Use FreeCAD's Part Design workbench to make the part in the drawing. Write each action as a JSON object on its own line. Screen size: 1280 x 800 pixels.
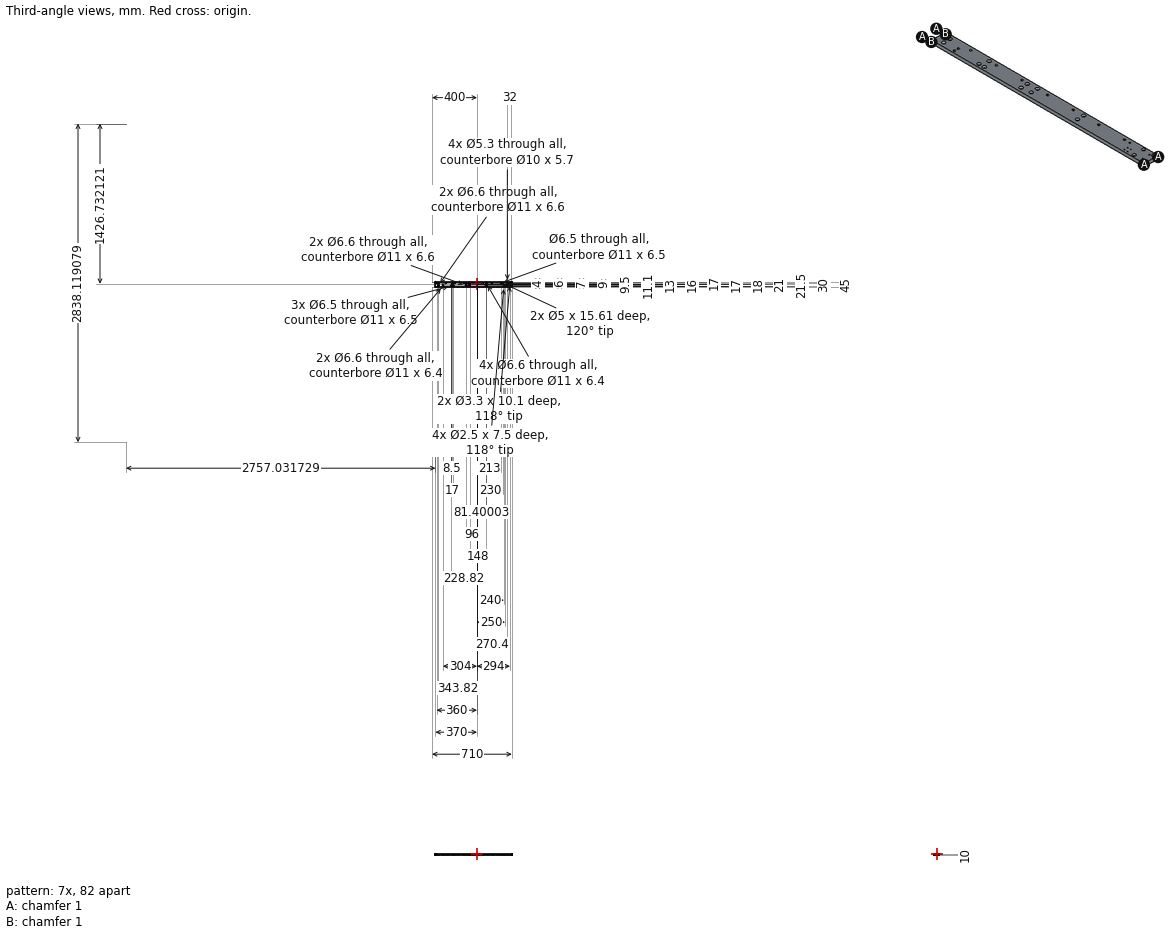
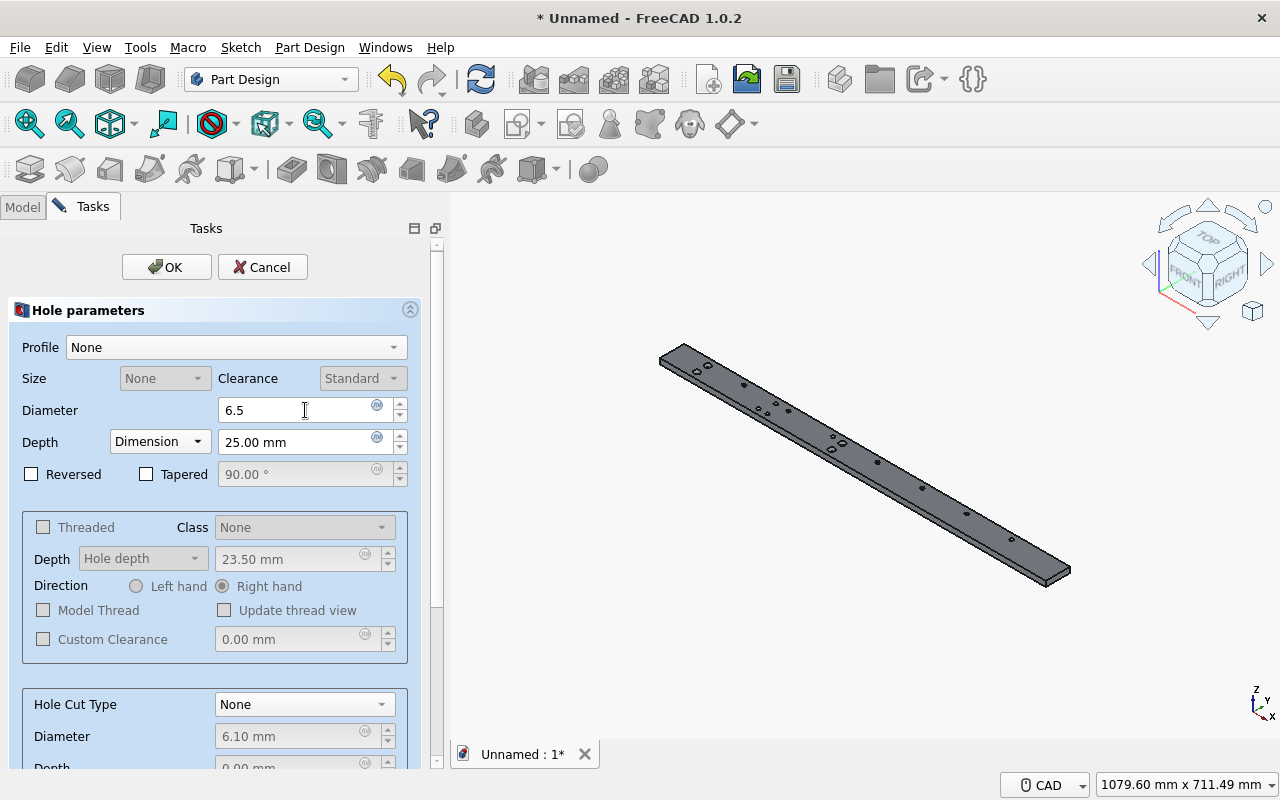
{"action": "left_click", "coordinate": [161, 442]}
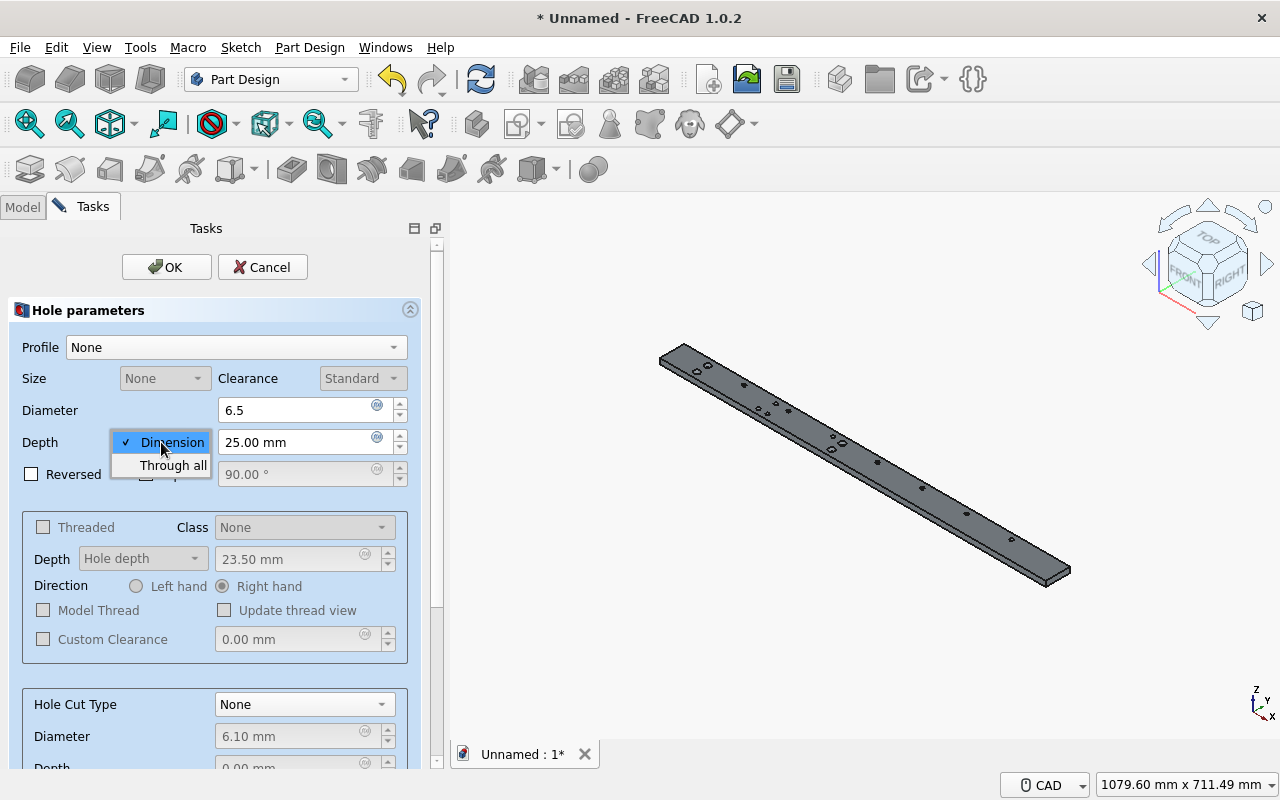
{"action": "left_click", "coordinate": [160, 466]}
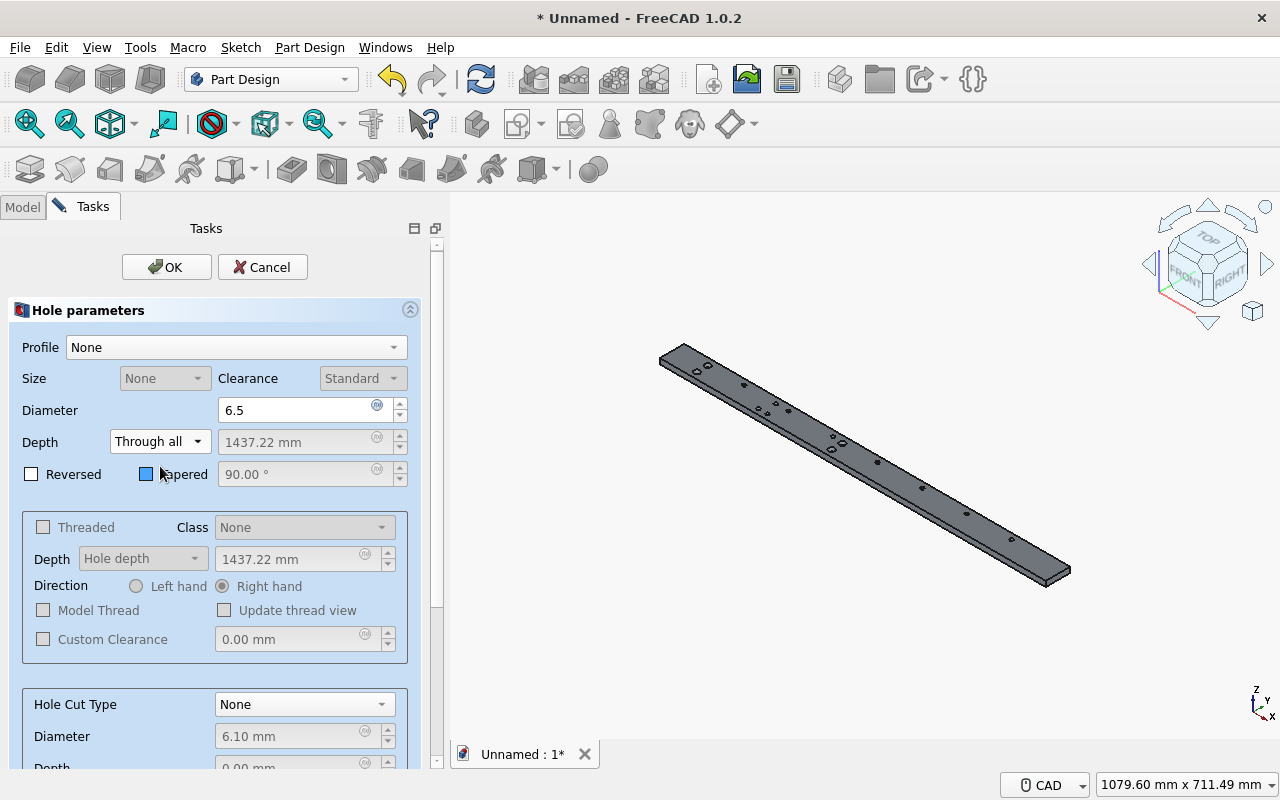
{"action": "left_click", "coordinate": [306, 704]}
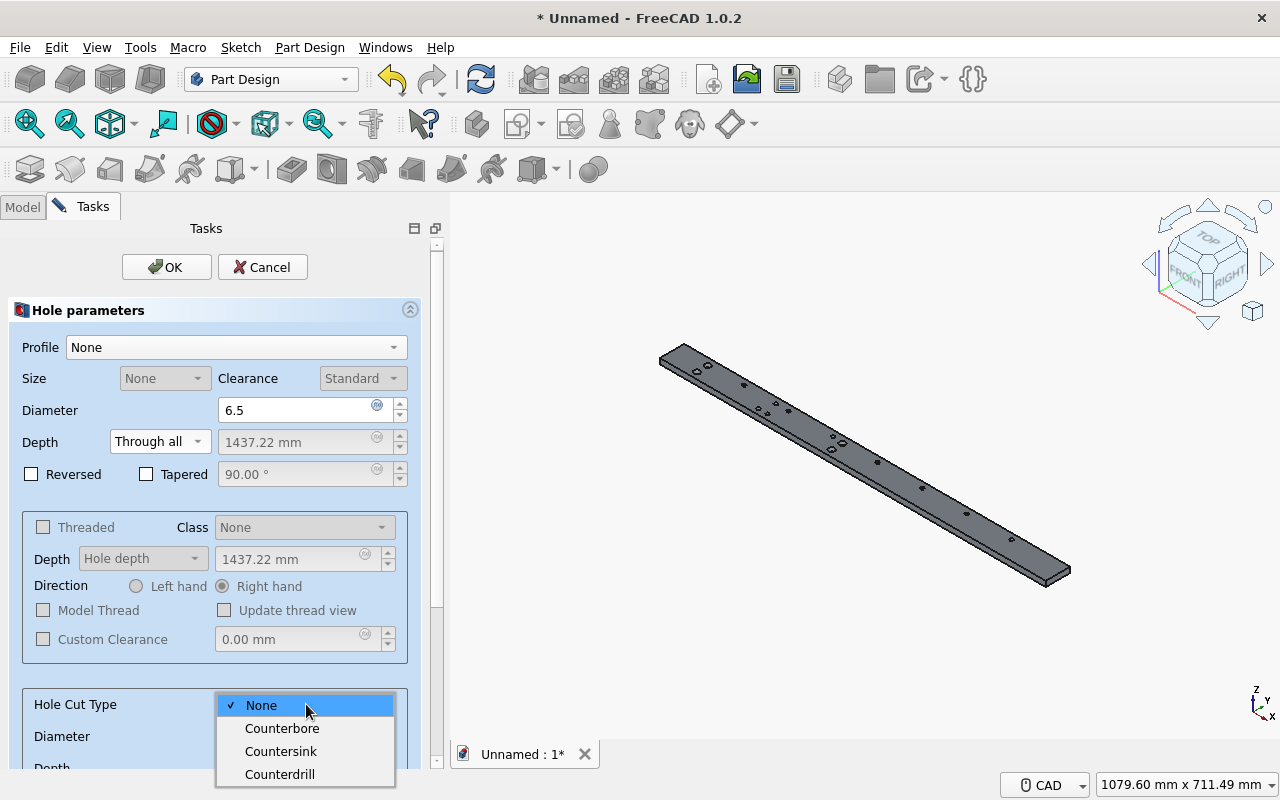
{"action": "left_click", "coordinate": [304, 728]}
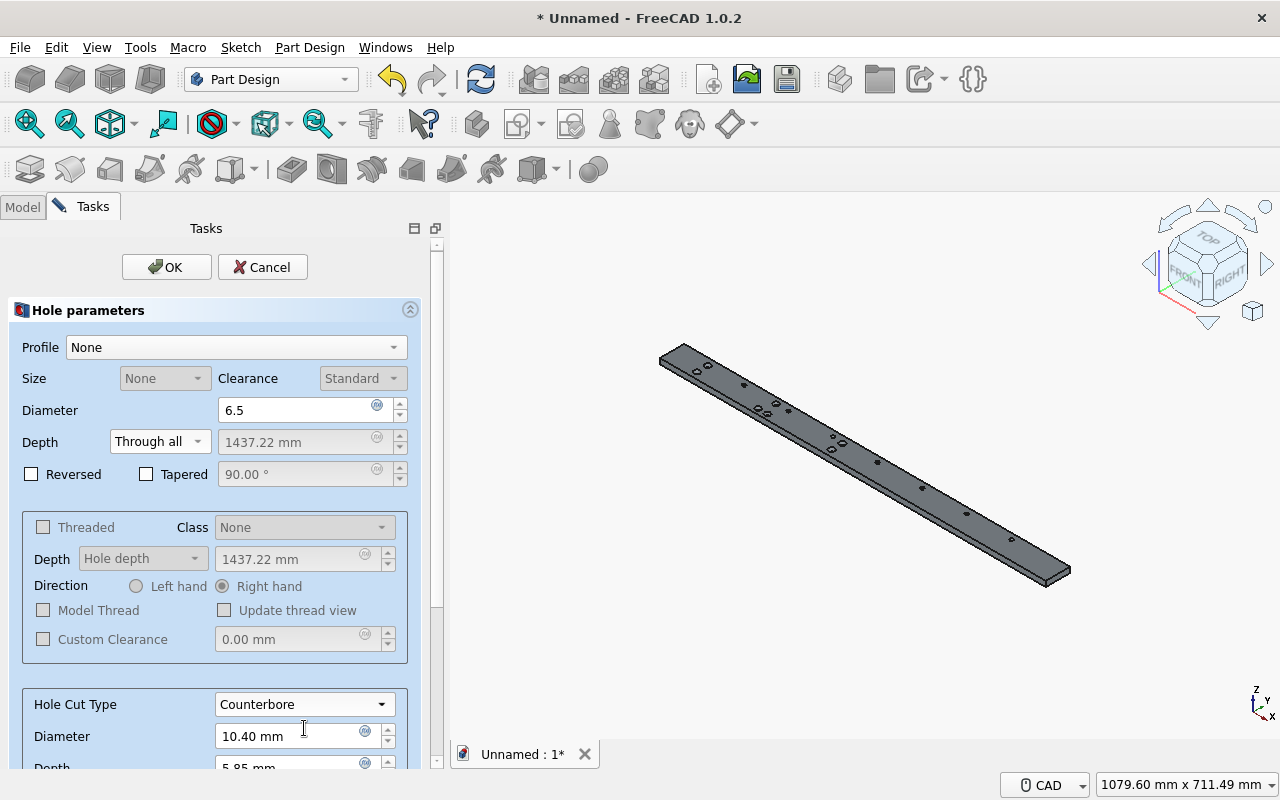
{"action": "triple_click", "coordinate": [298, 736]}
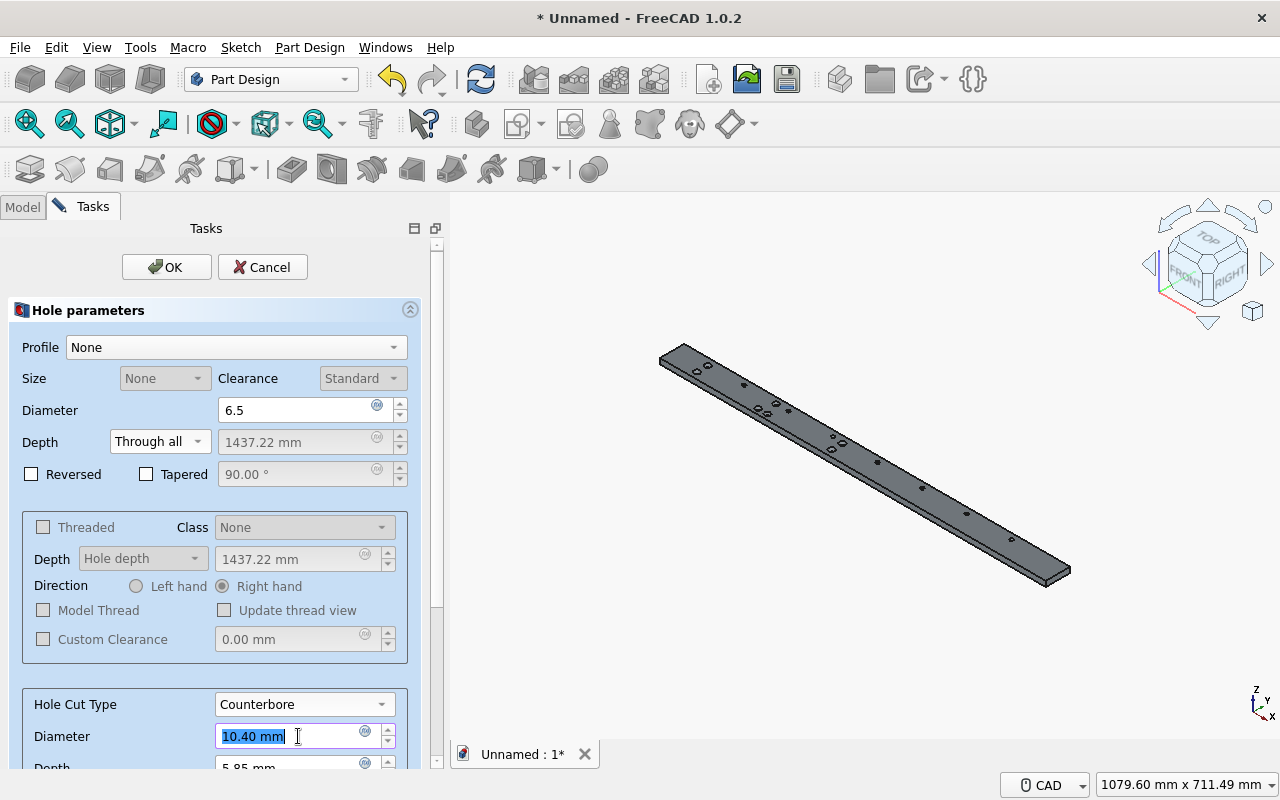
{"action": "type", "text": "11"}
{"action": "key", "text": "Tab"}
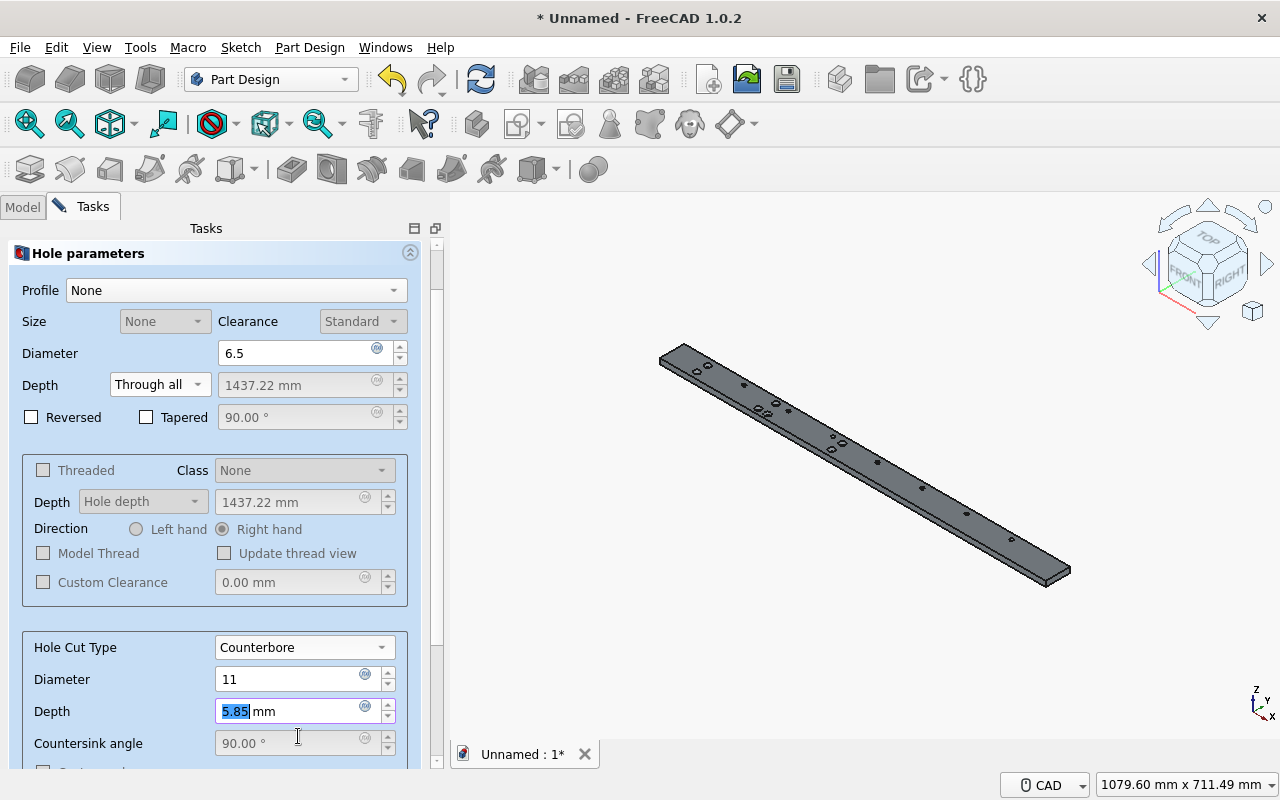
{"action": "type", "text": "6.5"}
{"action": "key", "text": "Tab"}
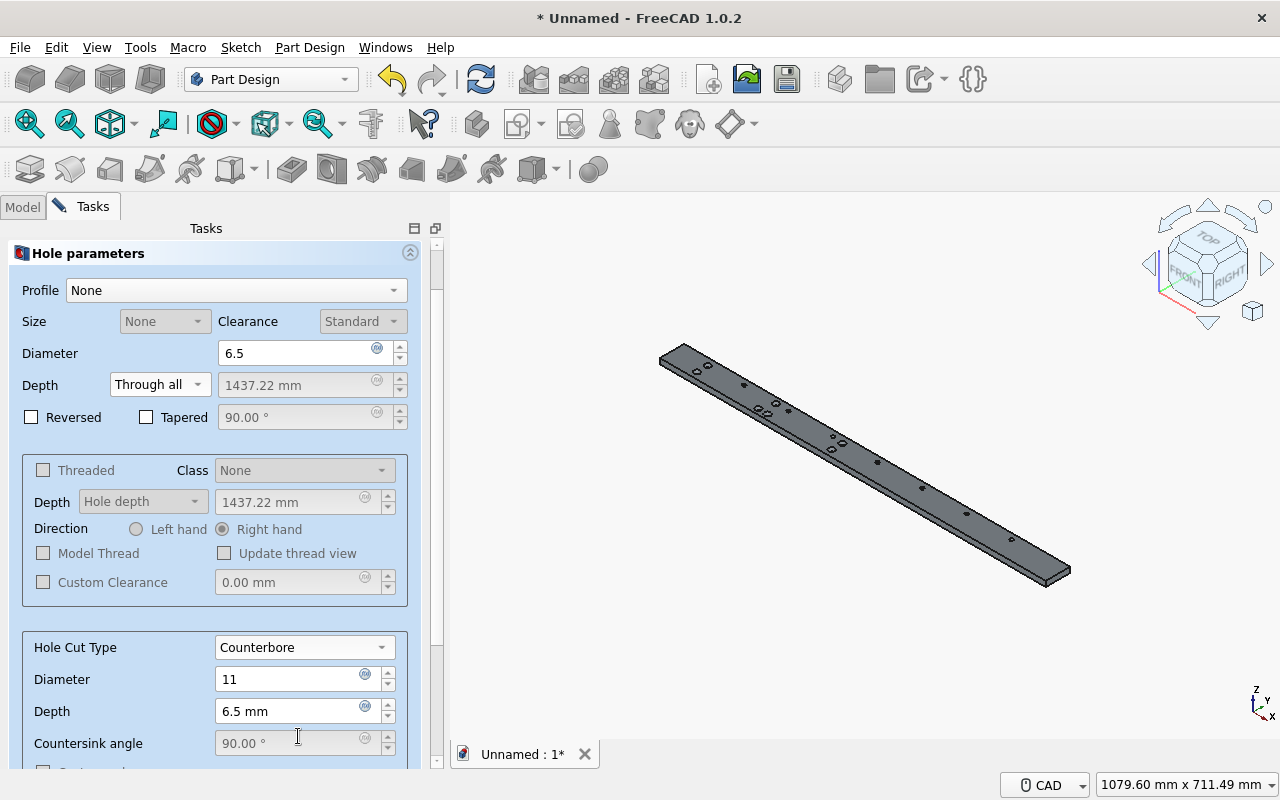
{"action": "scroll", "coordinate": [437, 503], "scroll_direction": "up", "scroll_amount": 2}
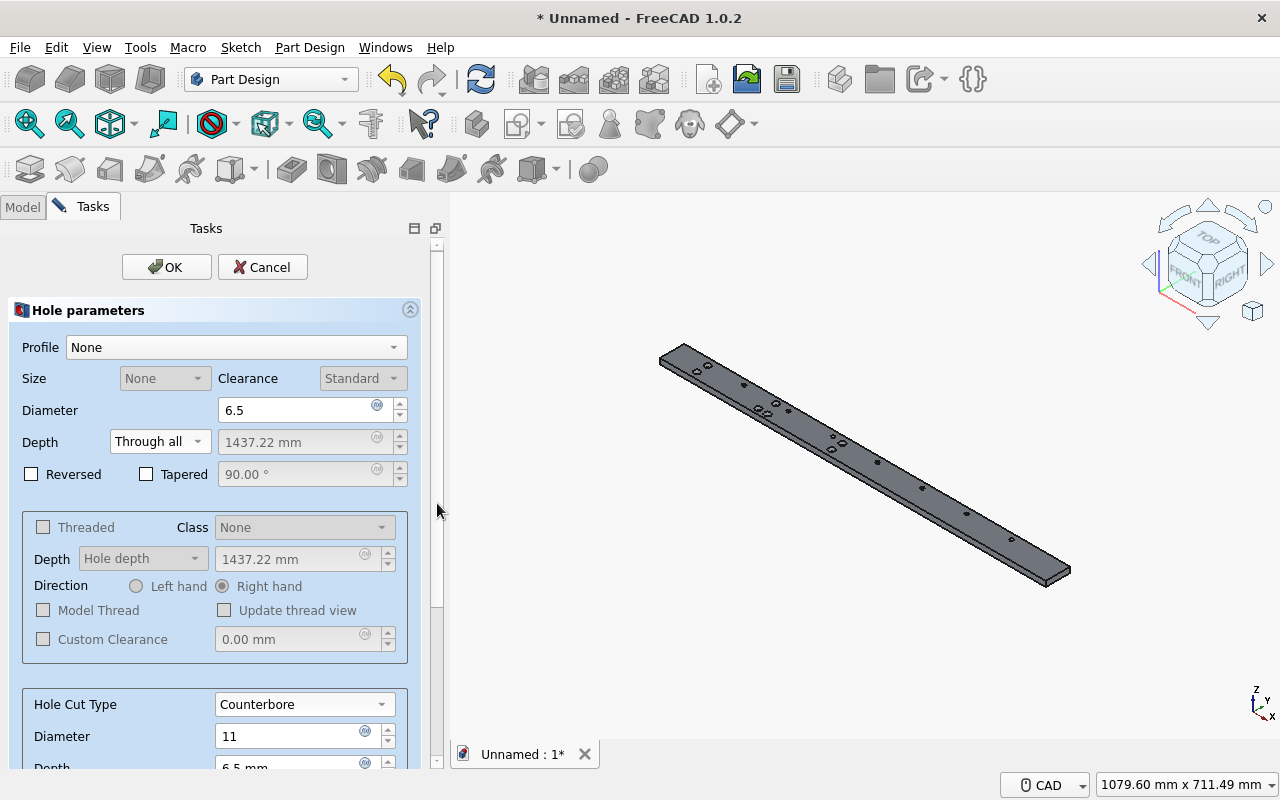
{"action": "left_click", "coordinate": [167, 267]}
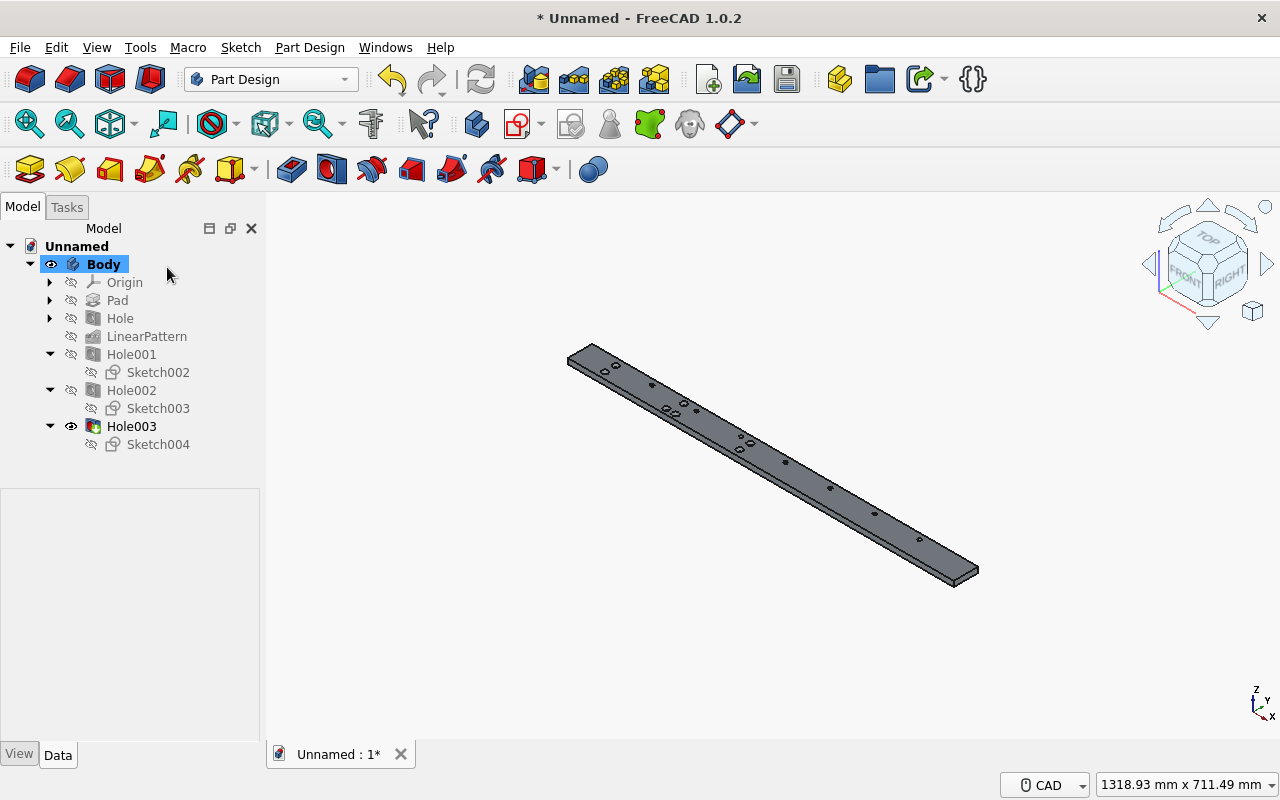
{"action": "left_click", "coordinate": [30, 124]}